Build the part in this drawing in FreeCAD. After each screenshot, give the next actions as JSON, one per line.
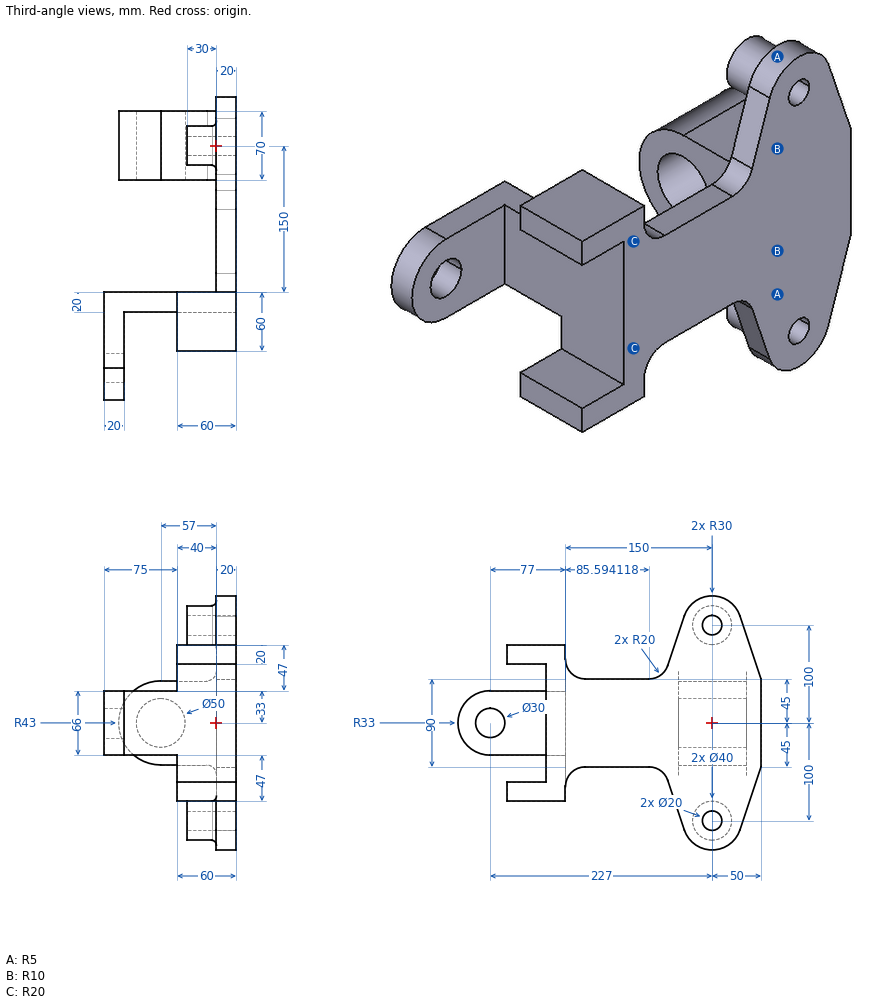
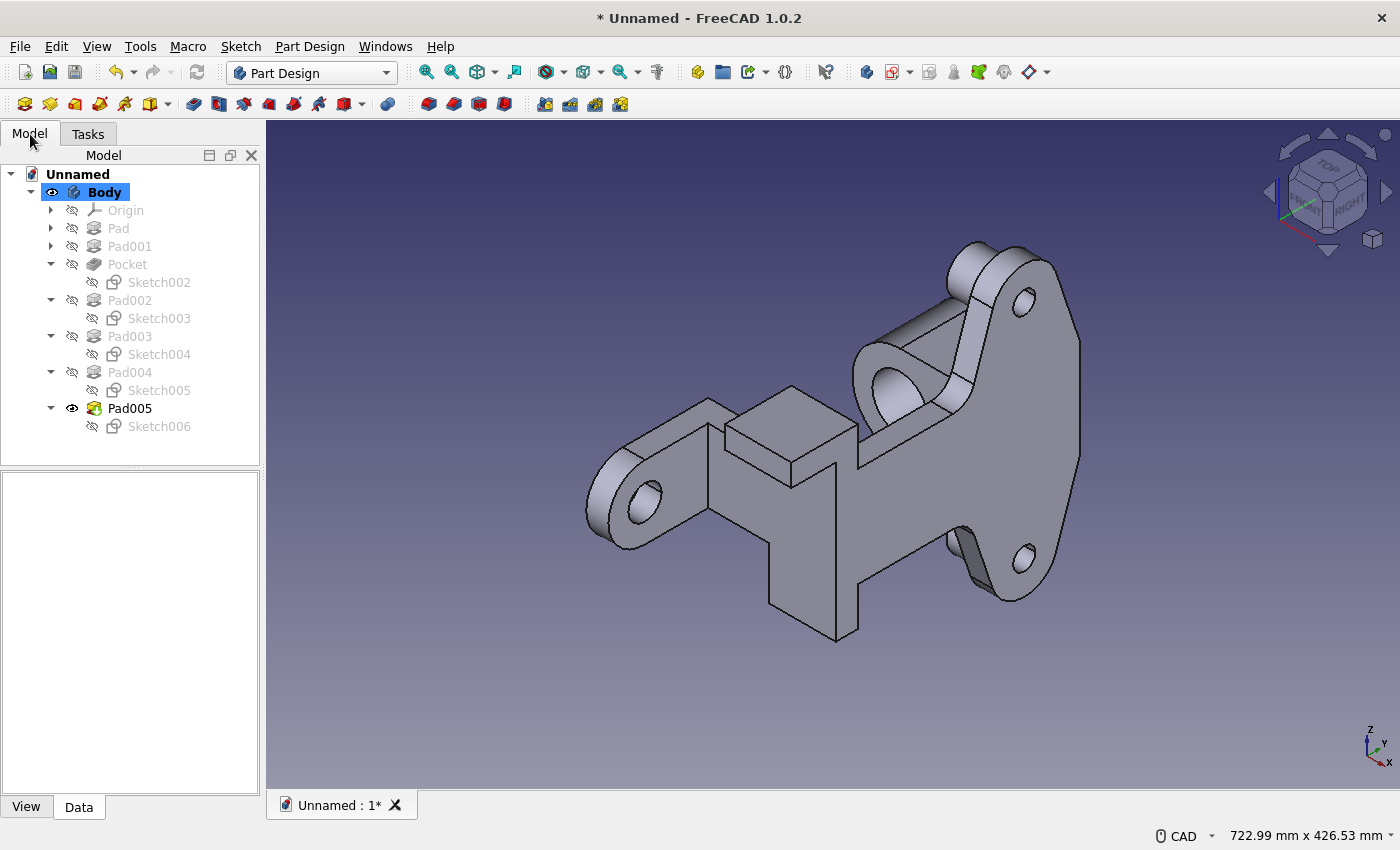
{"action": "left_click", "coordinate": [117, 408]}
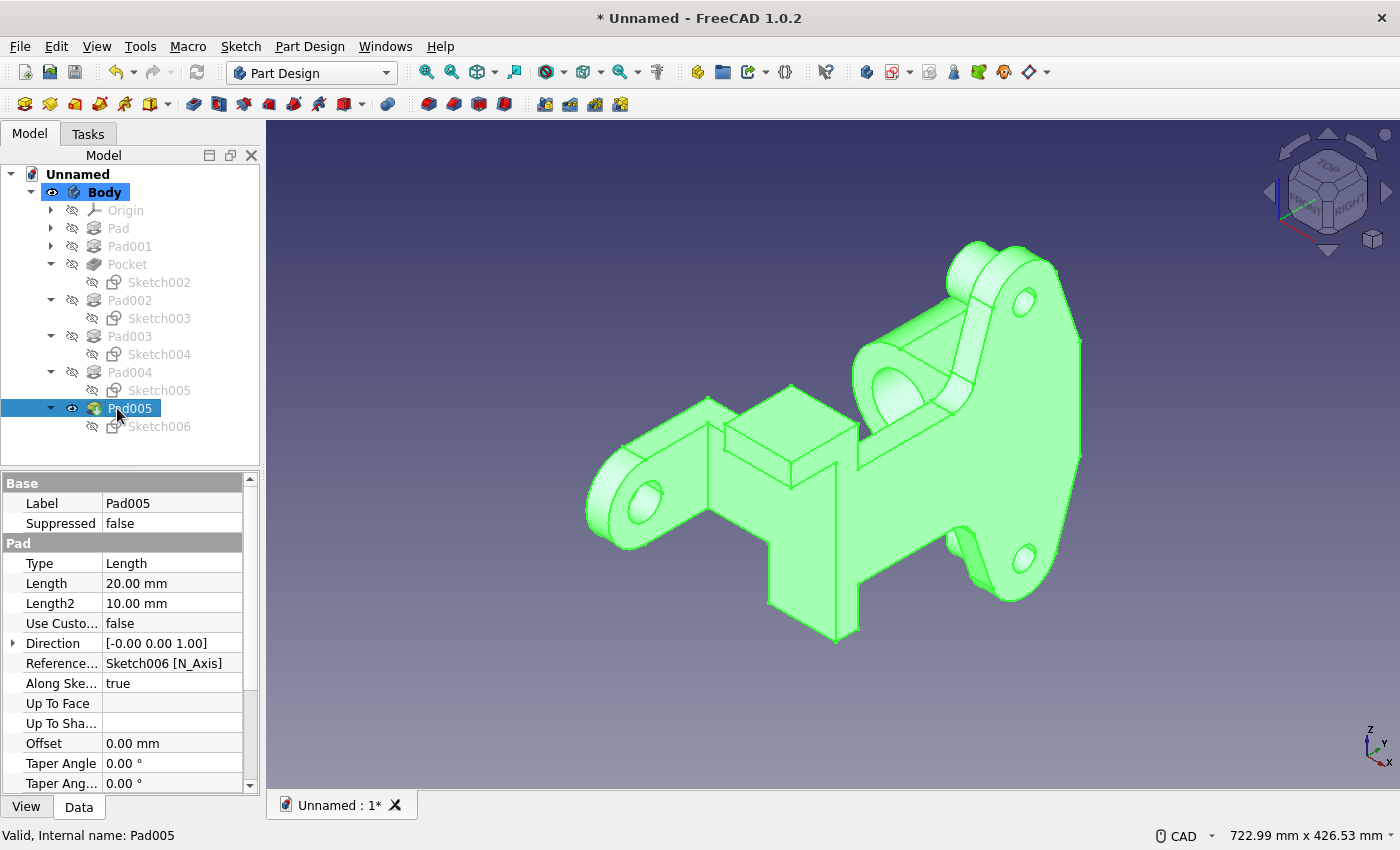
{"action": "left_click", "coordinate": [545, 104]}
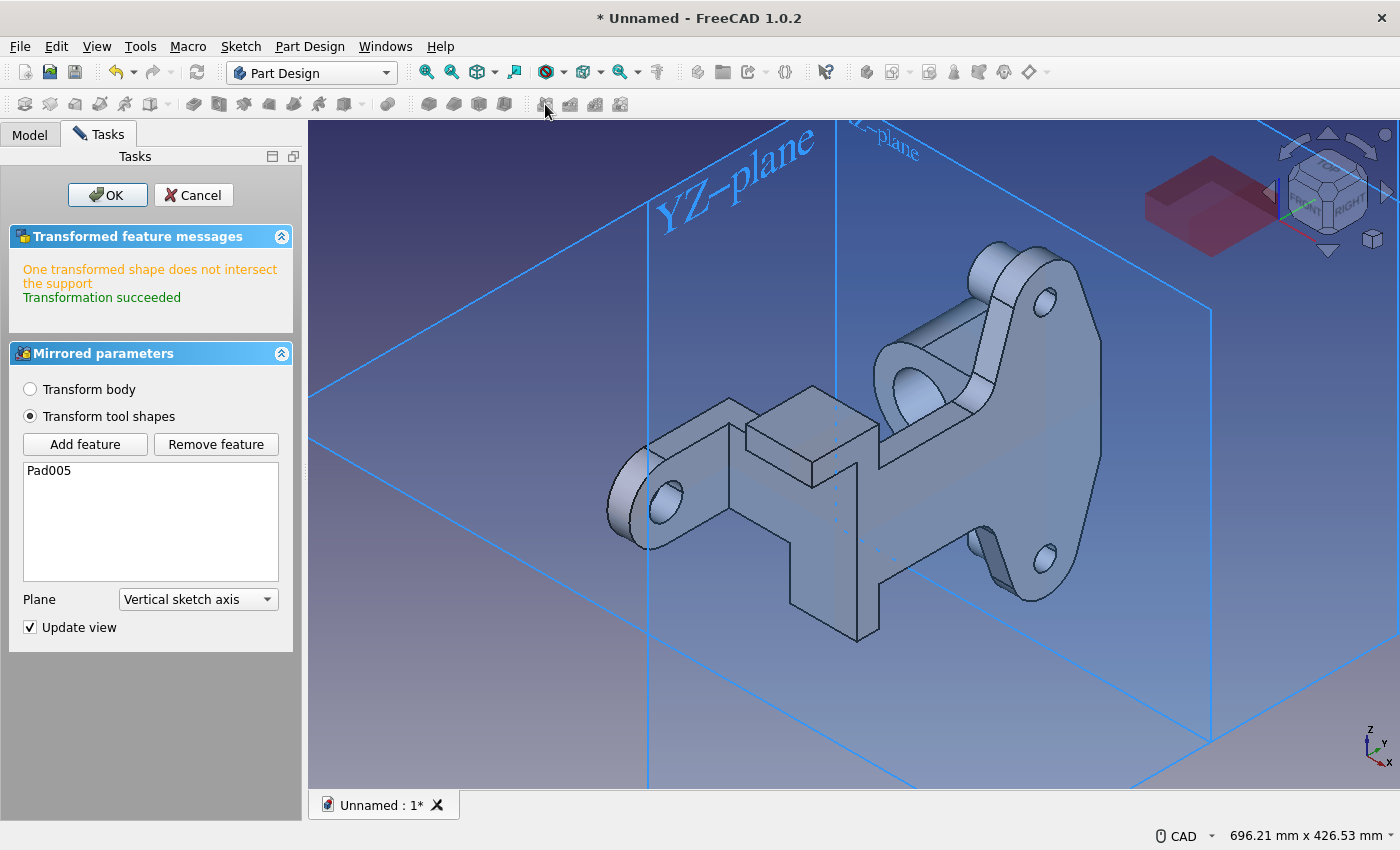
{"action": "left_click", "coordinate": [199, 600]}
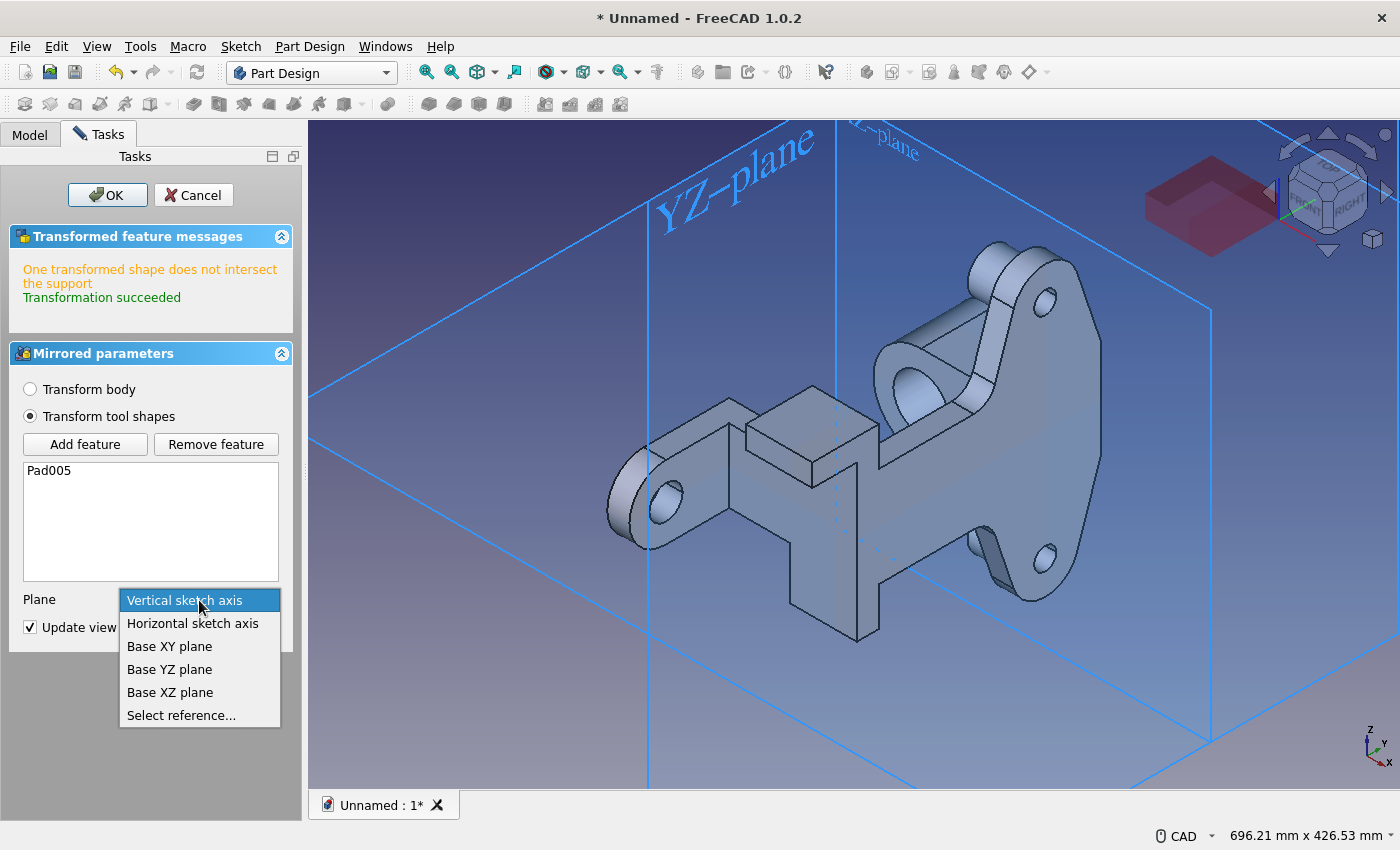
{"action": "left_click", "coordinate": [198, 646]}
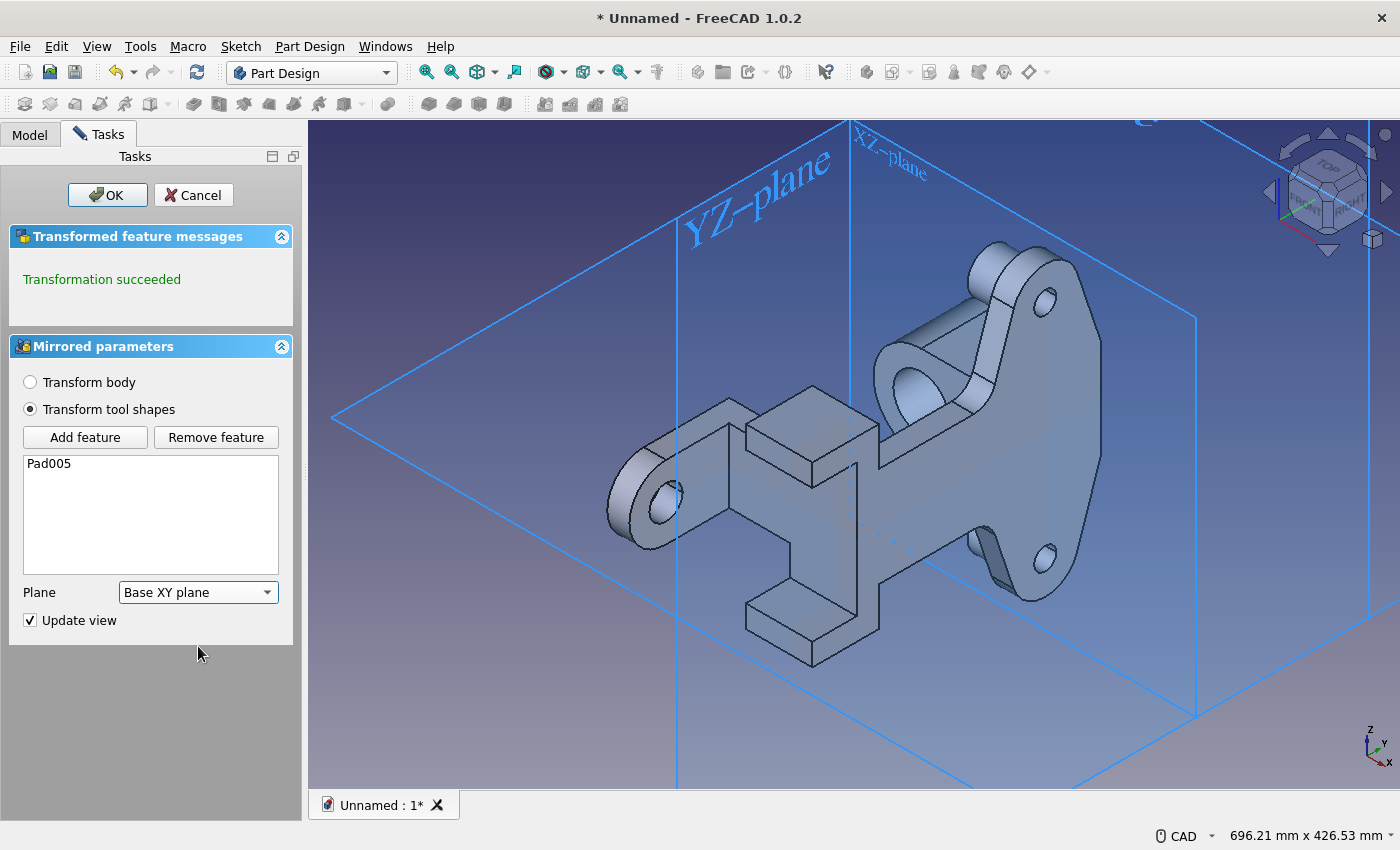
{"action": "left_click", "coordinate": [108, 195]}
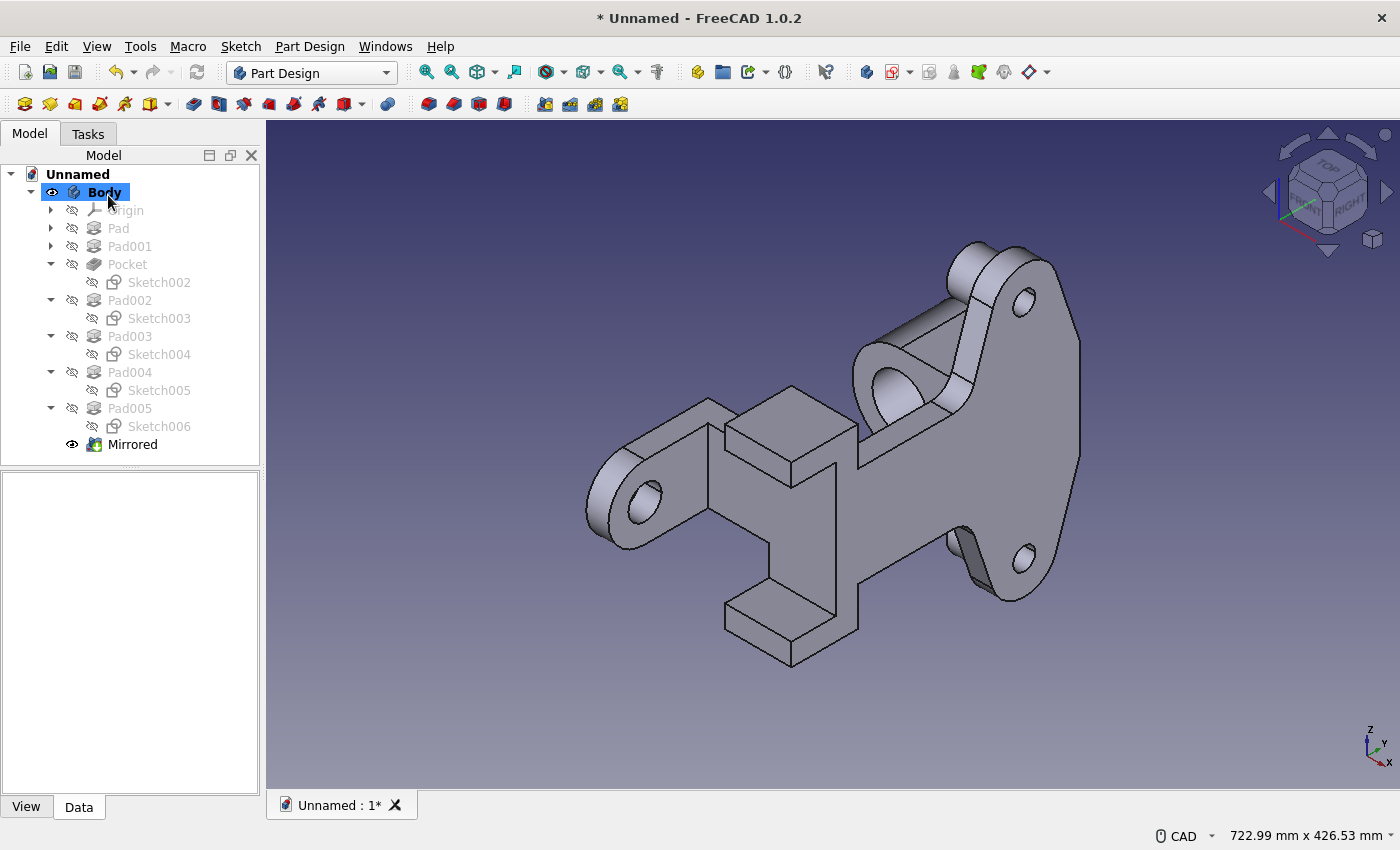
{"action": "key", "text": "2"}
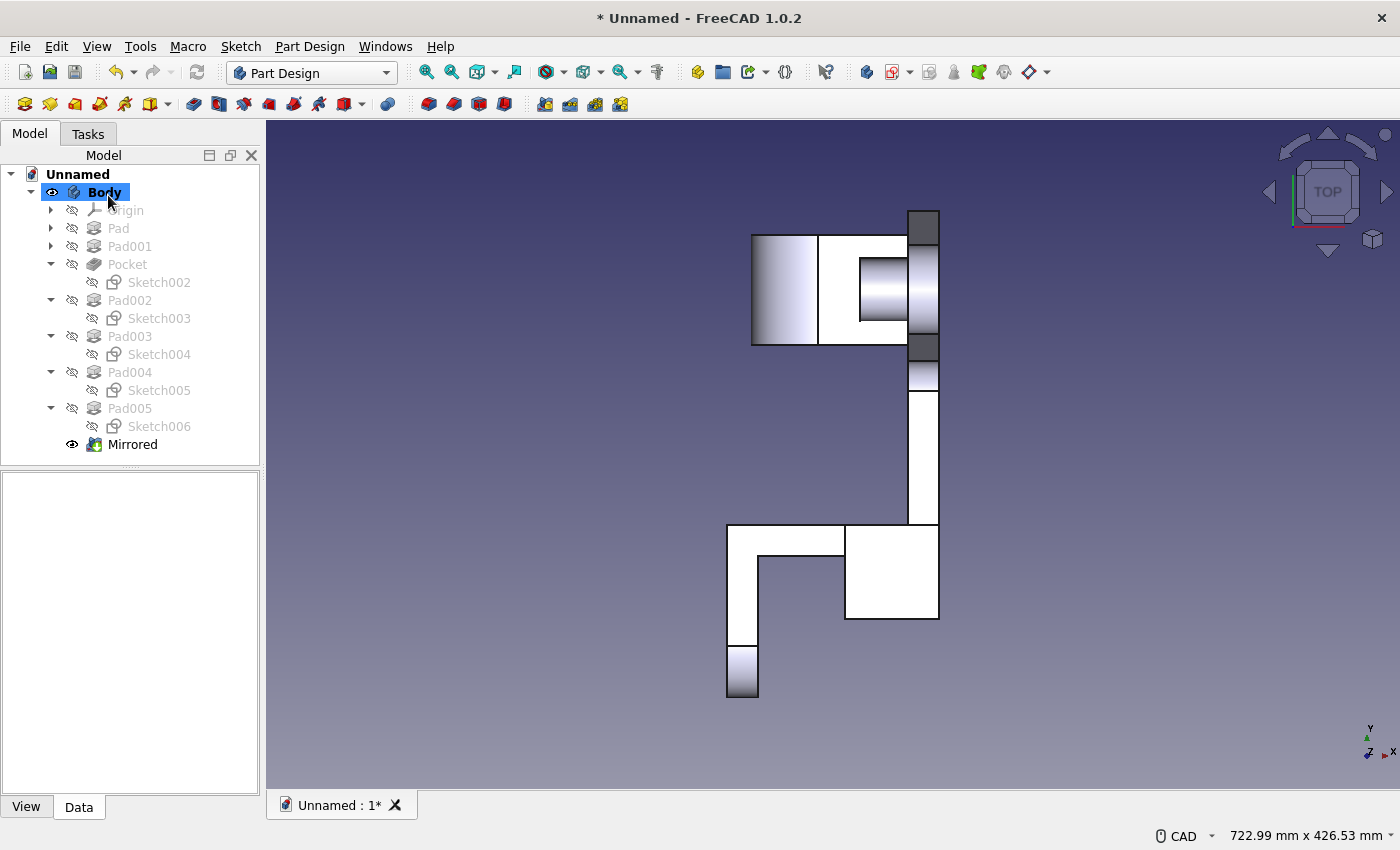
{"action": "key", "text": "0"}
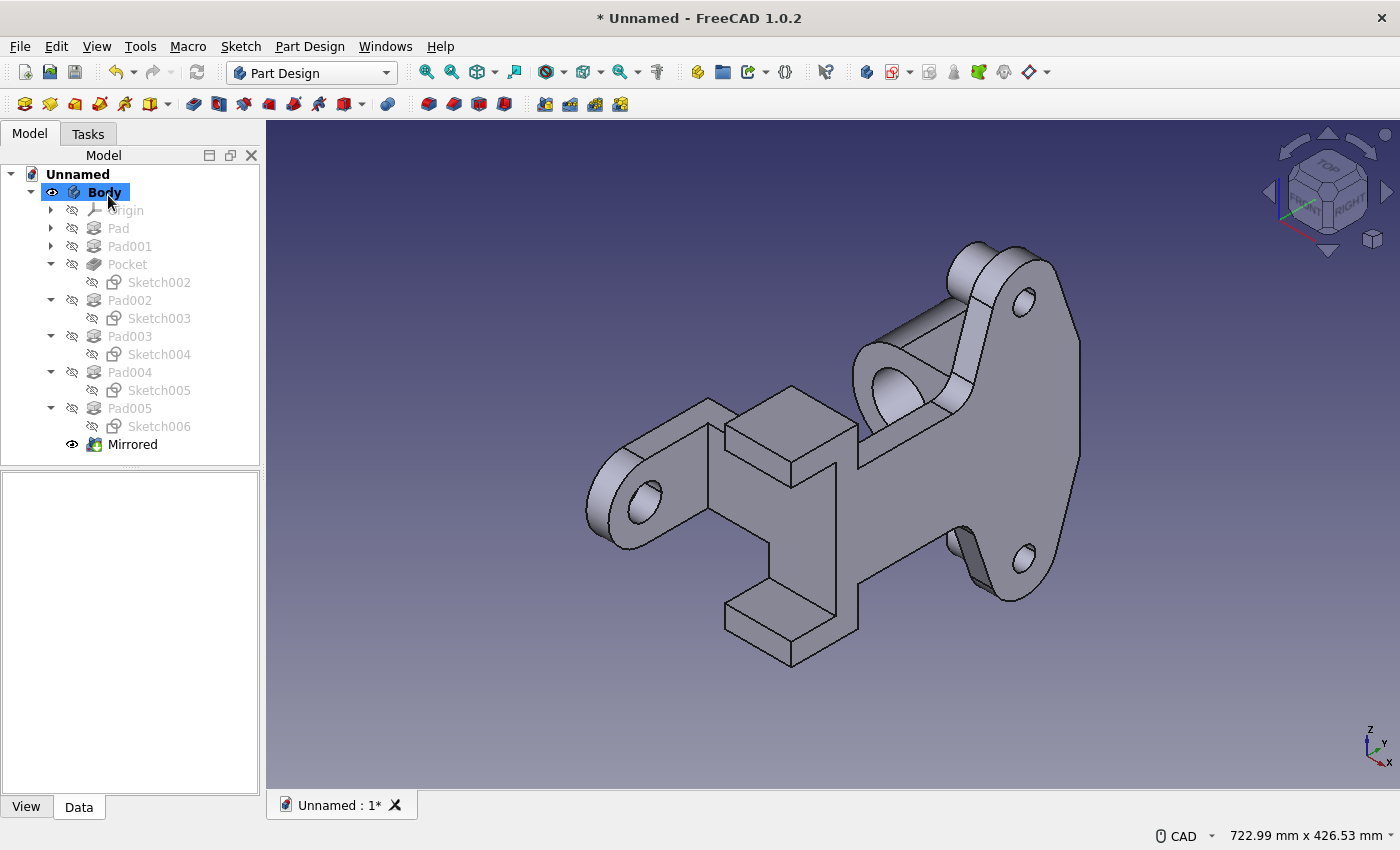
{"action": "key", "text": "1"}